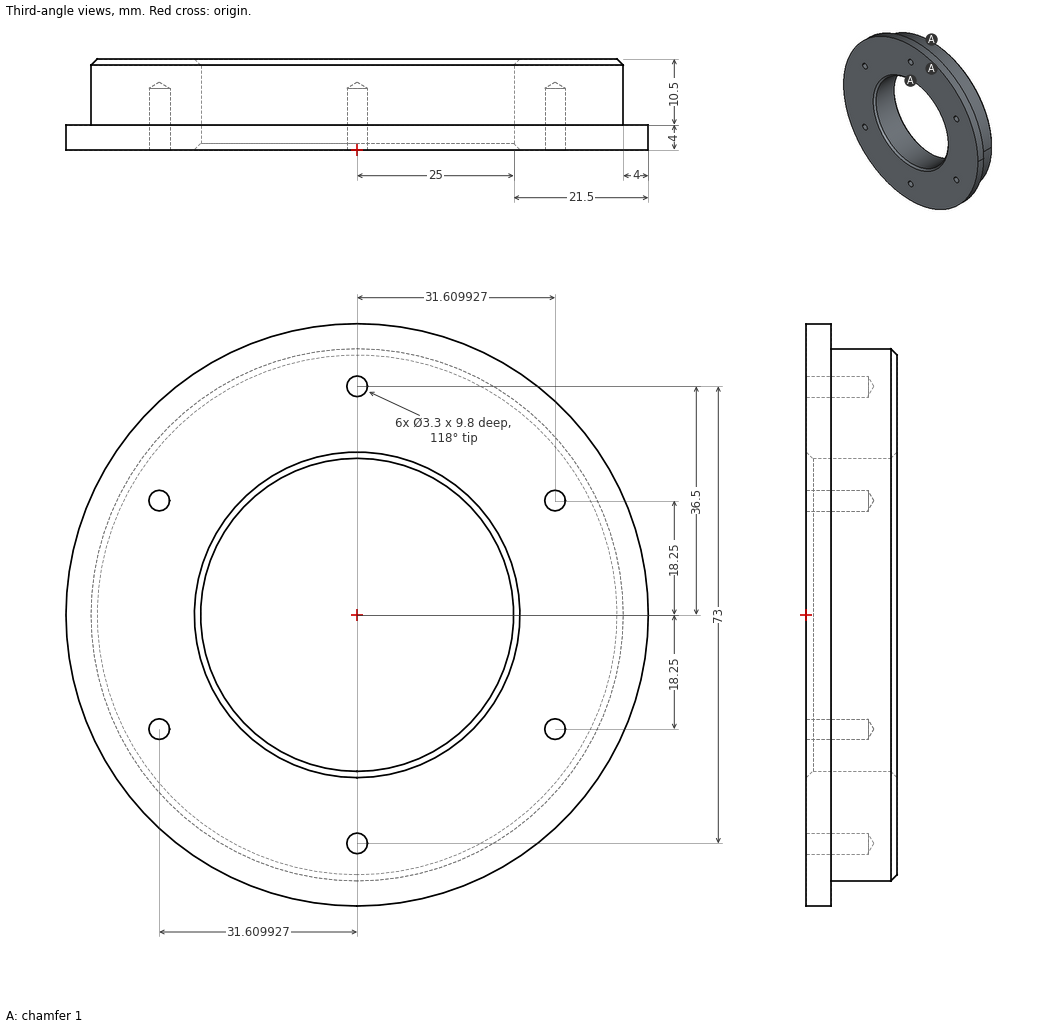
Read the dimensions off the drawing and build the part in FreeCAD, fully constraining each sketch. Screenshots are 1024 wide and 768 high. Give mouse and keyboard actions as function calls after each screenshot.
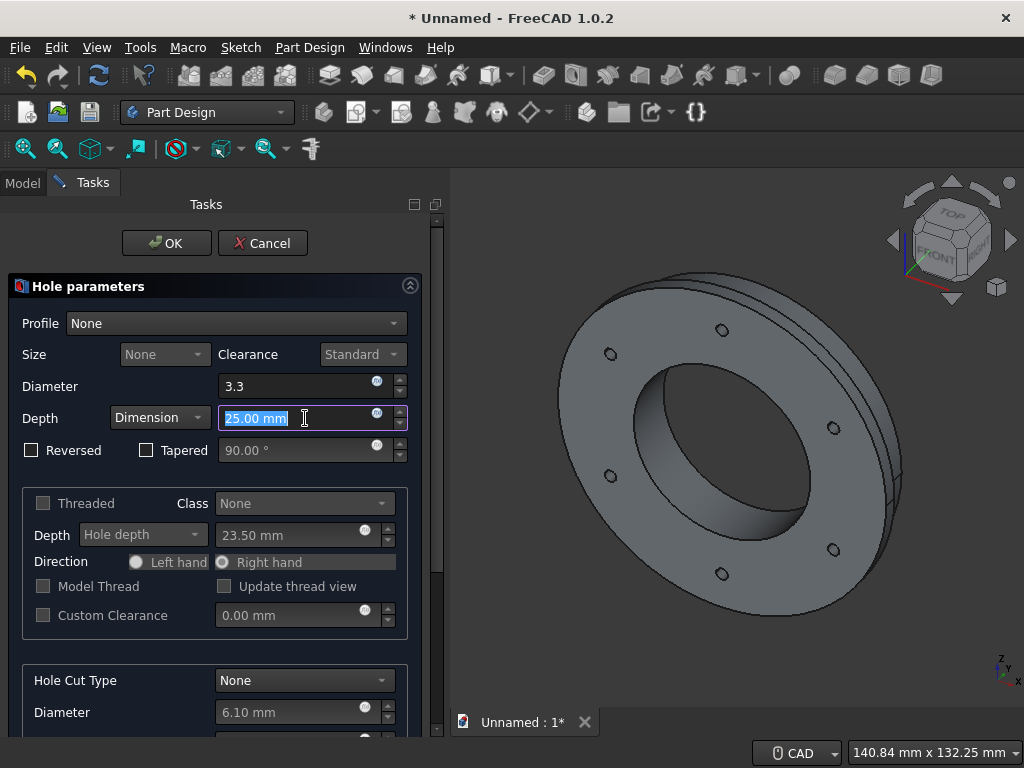
text(9.8)
key(Tab)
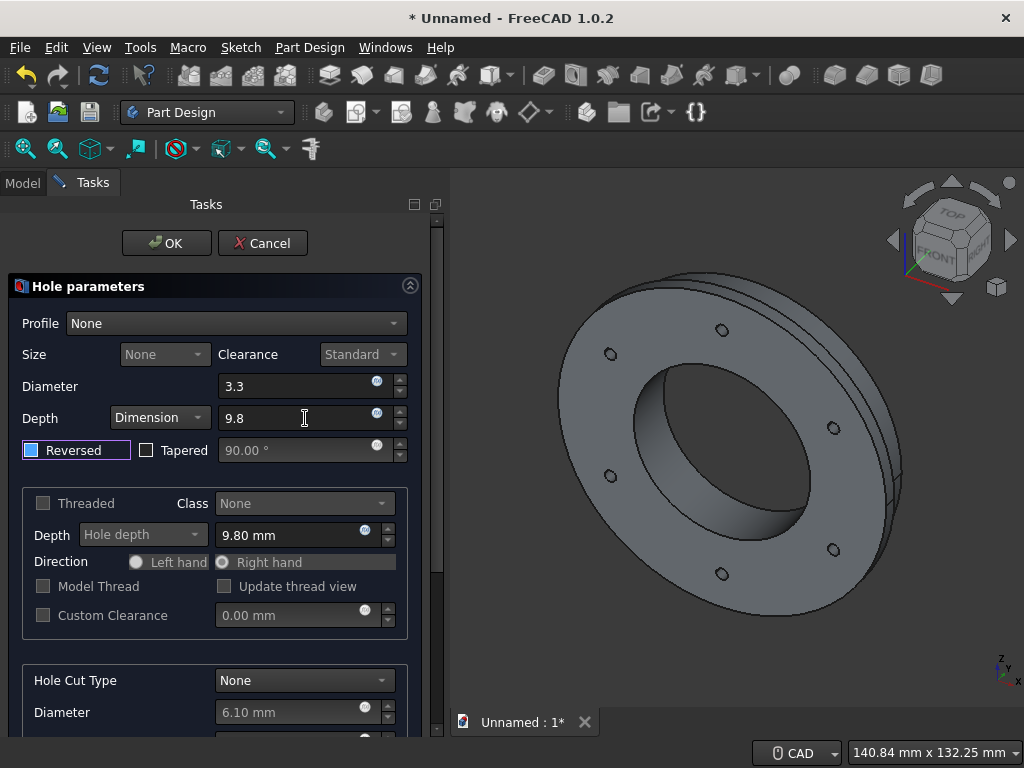
click(167, 243)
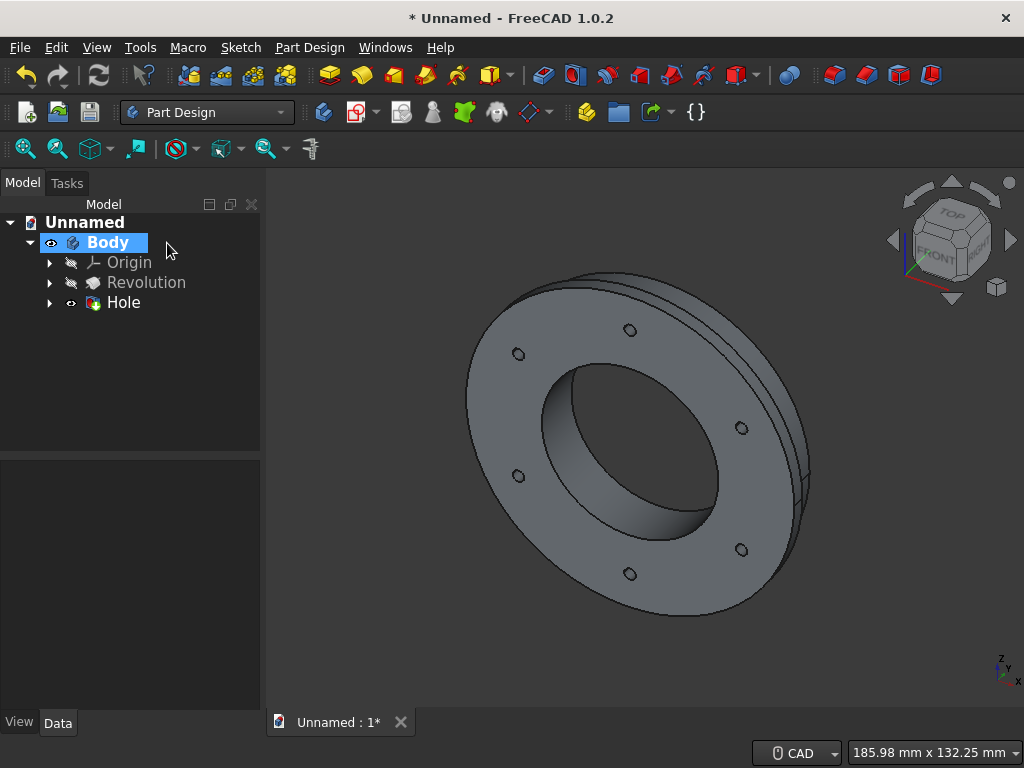
click(542, 422)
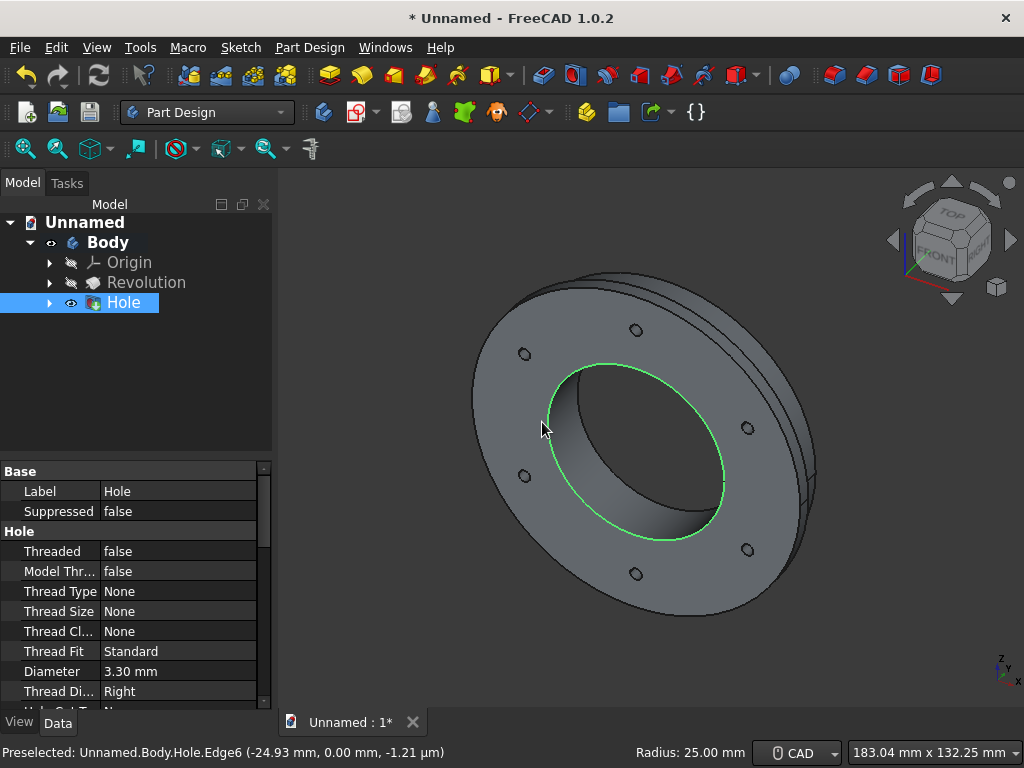
key(0)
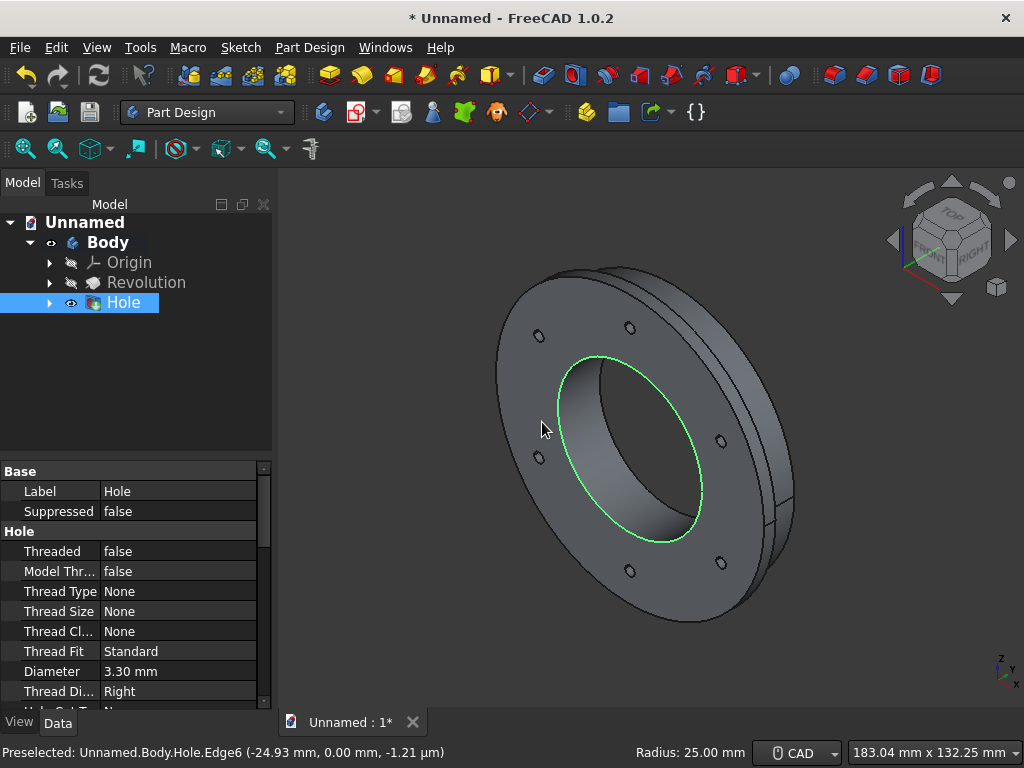
key(2)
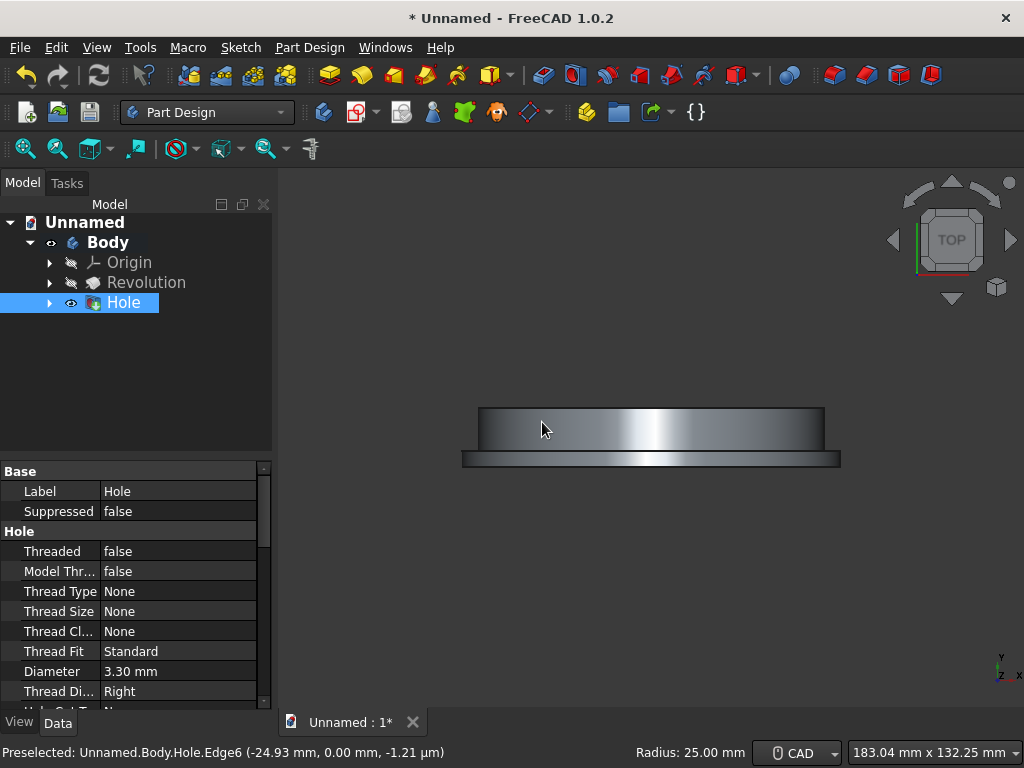
click(511, 407, ctrl)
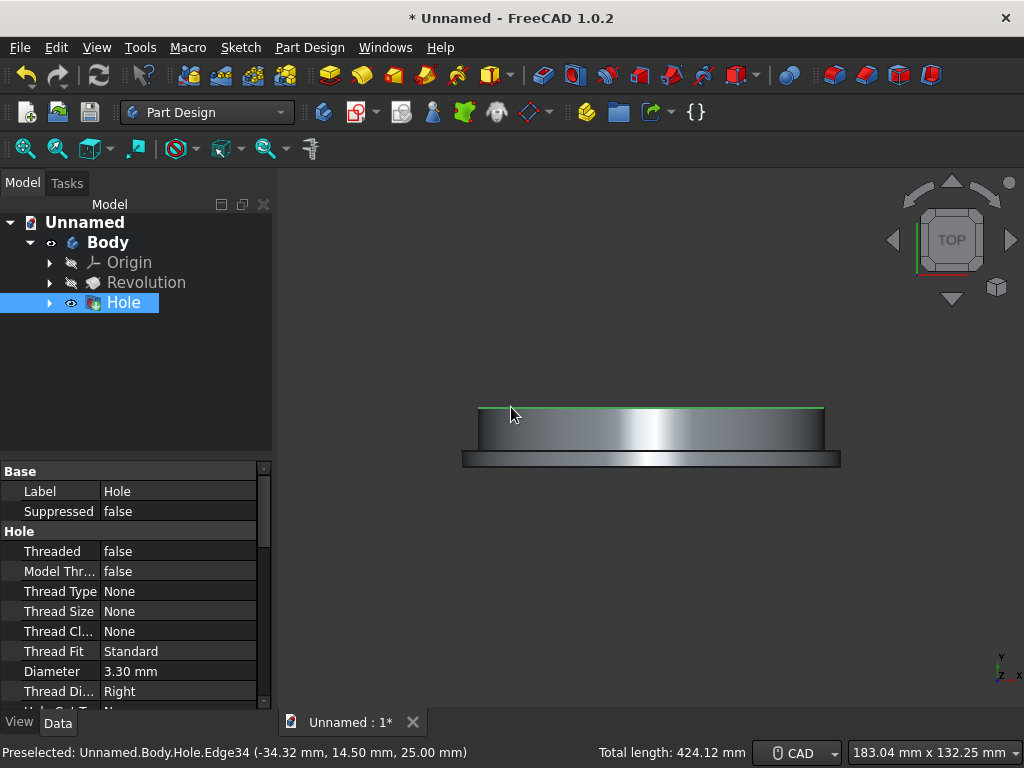
key(1)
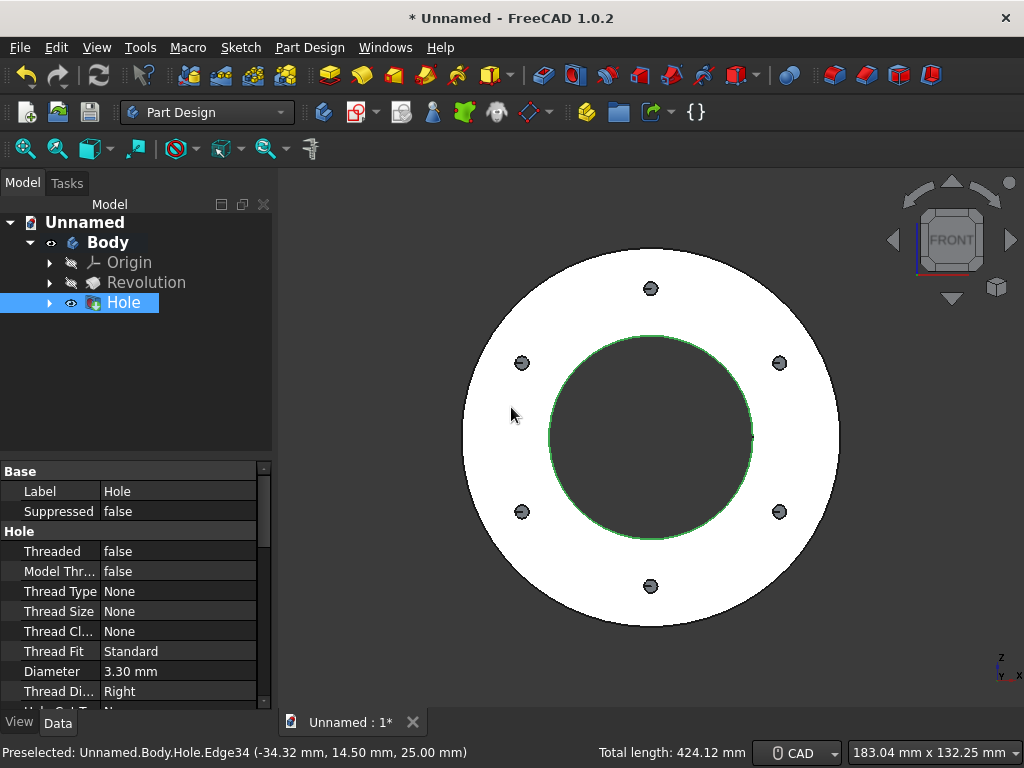
key(3)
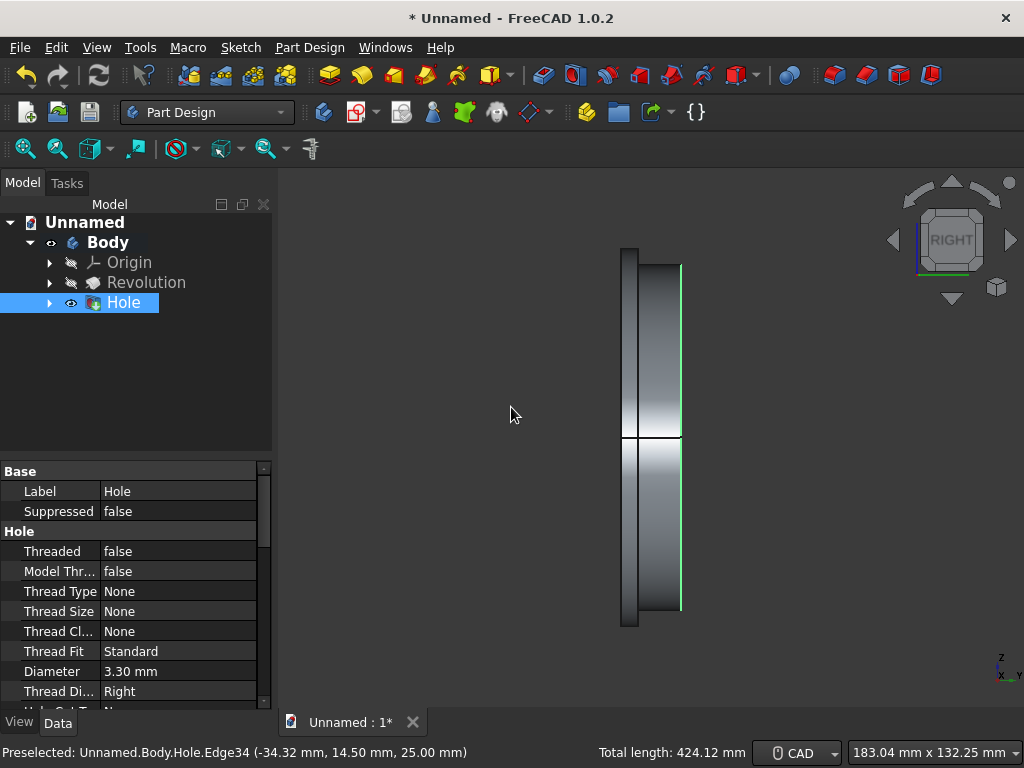
key(5)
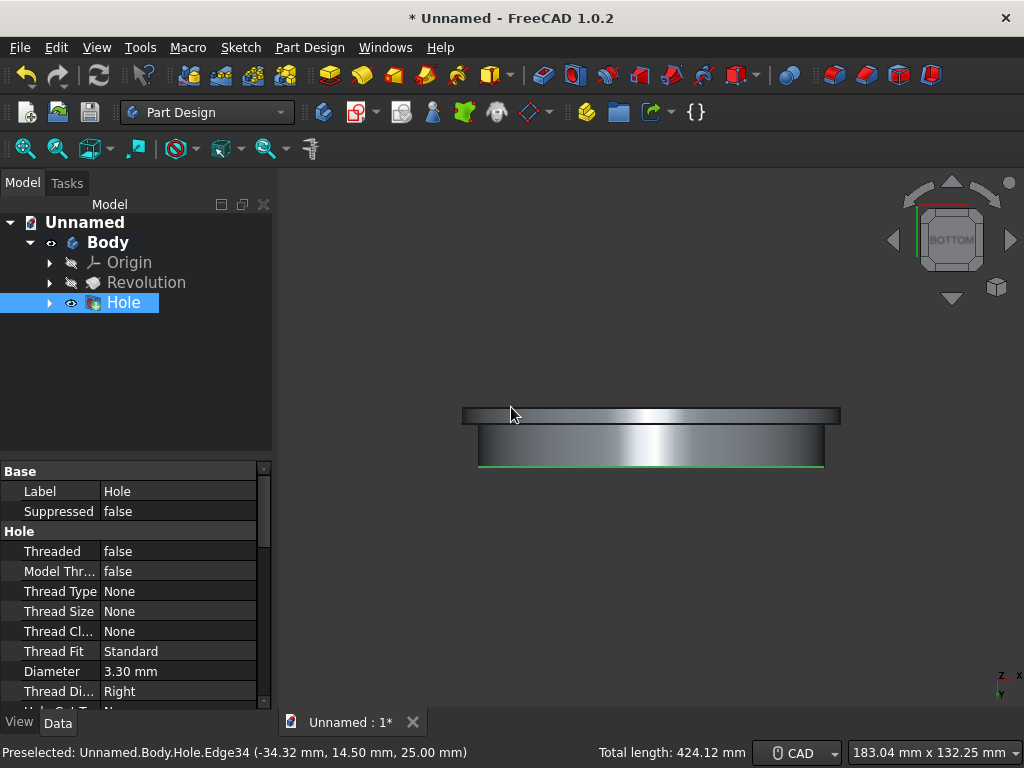
key(4)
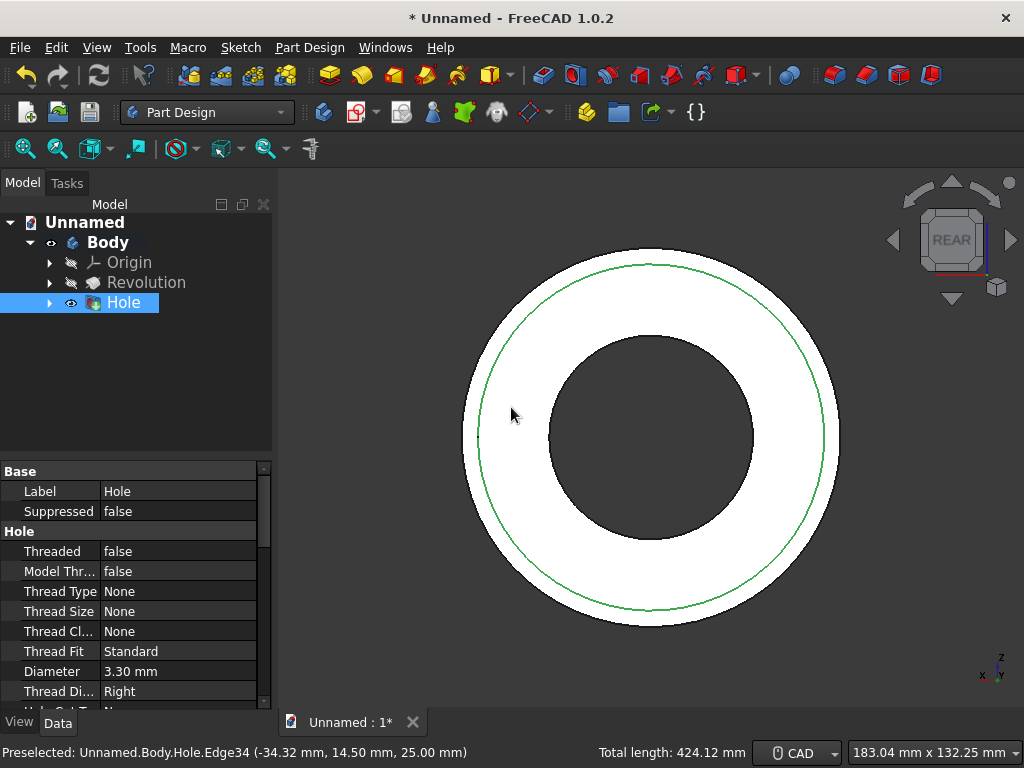
click(753, 436, ctrl)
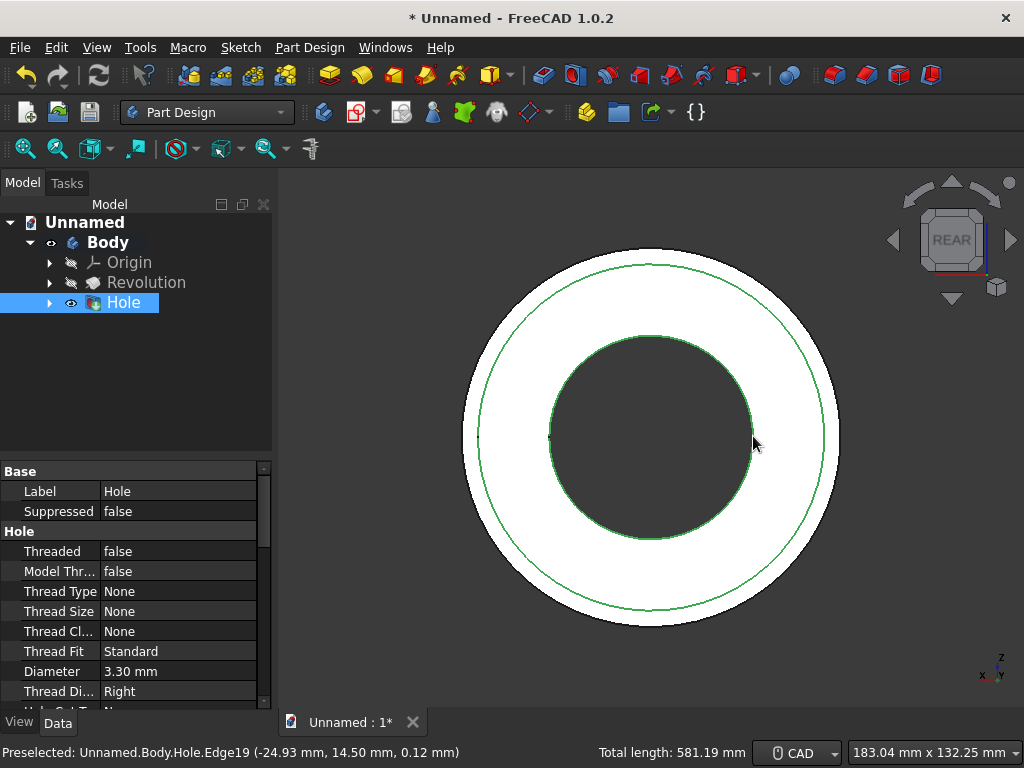
click(868, 76)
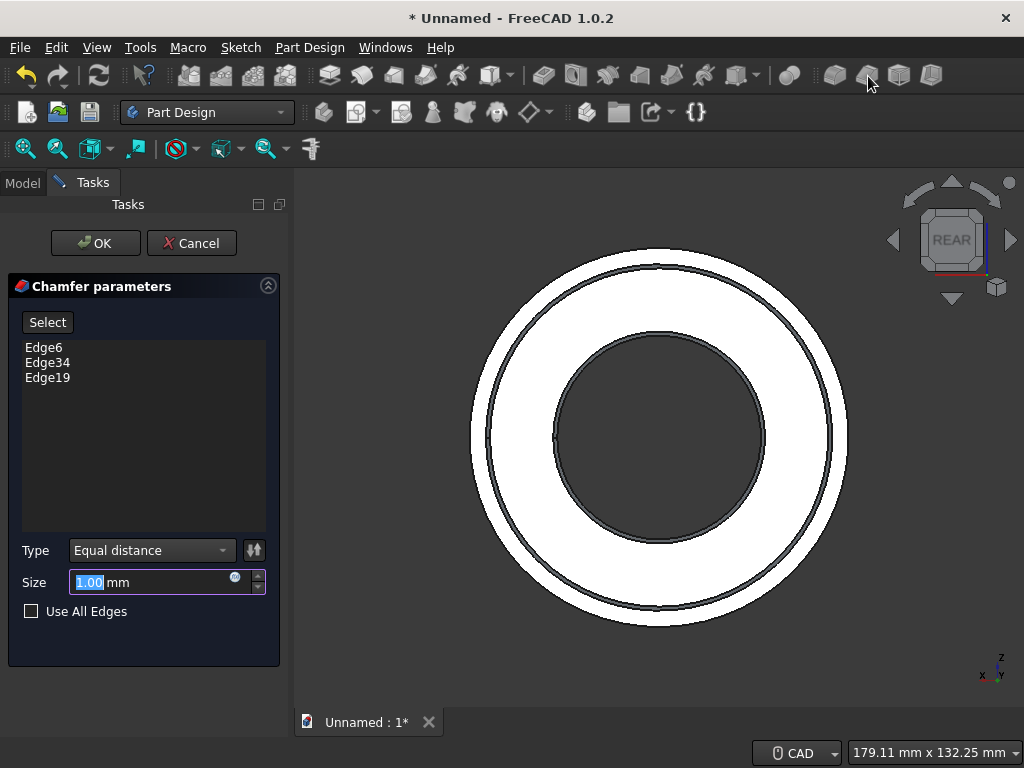
text(1)
key(Tab)